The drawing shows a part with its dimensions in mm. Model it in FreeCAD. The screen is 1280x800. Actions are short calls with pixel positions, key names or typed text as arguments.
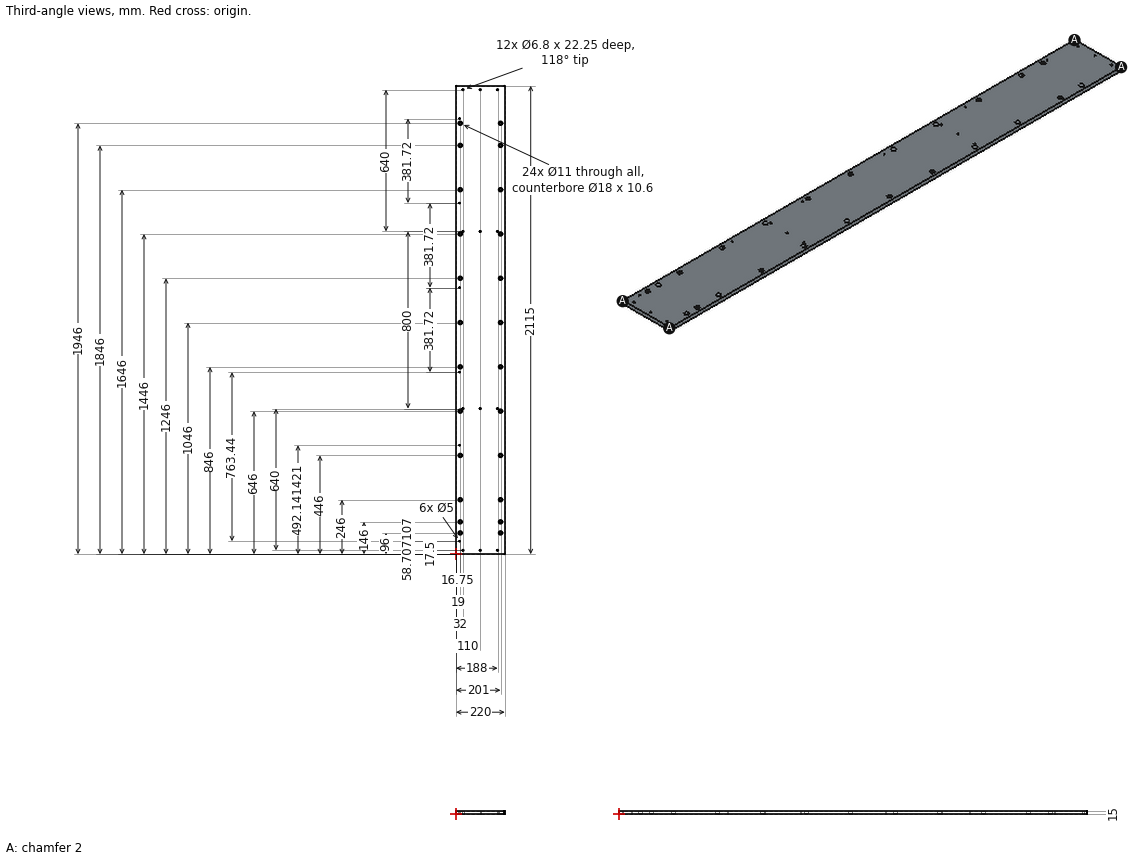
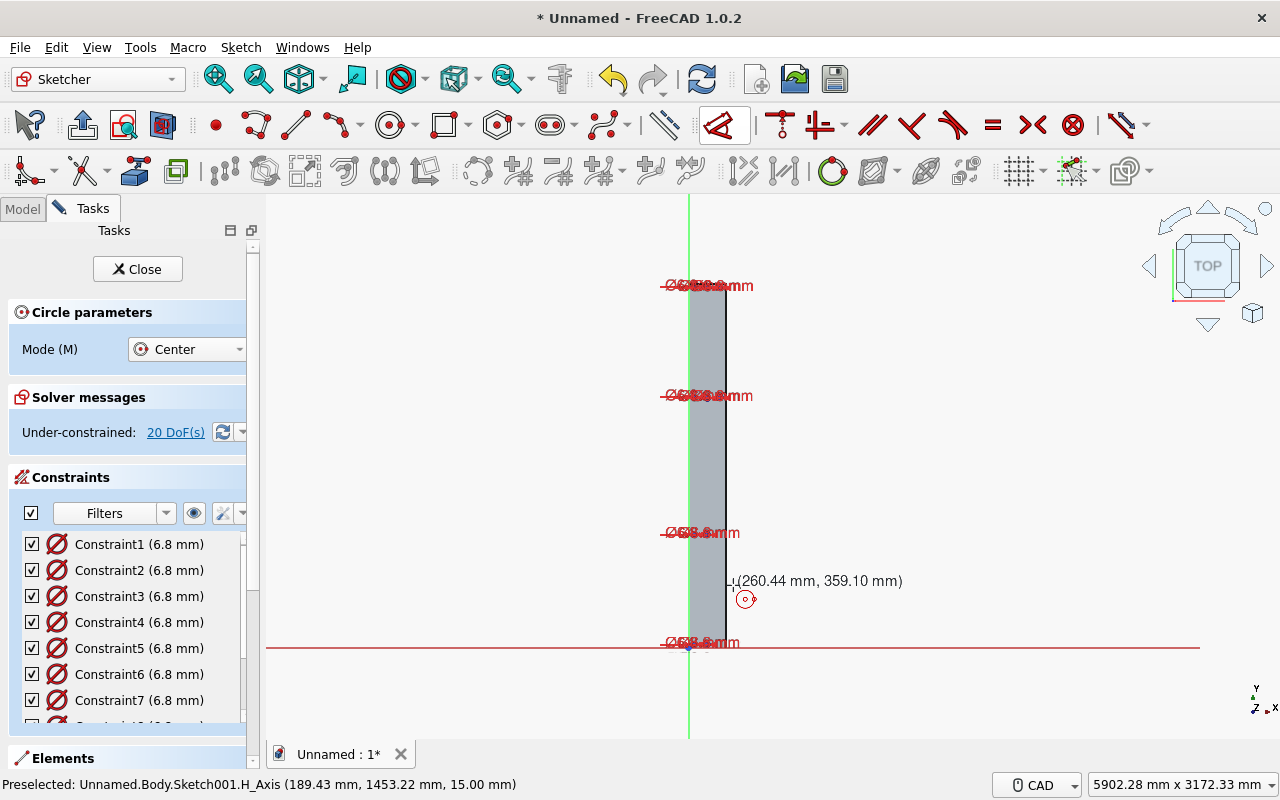
scroll(721, 535, up, 2)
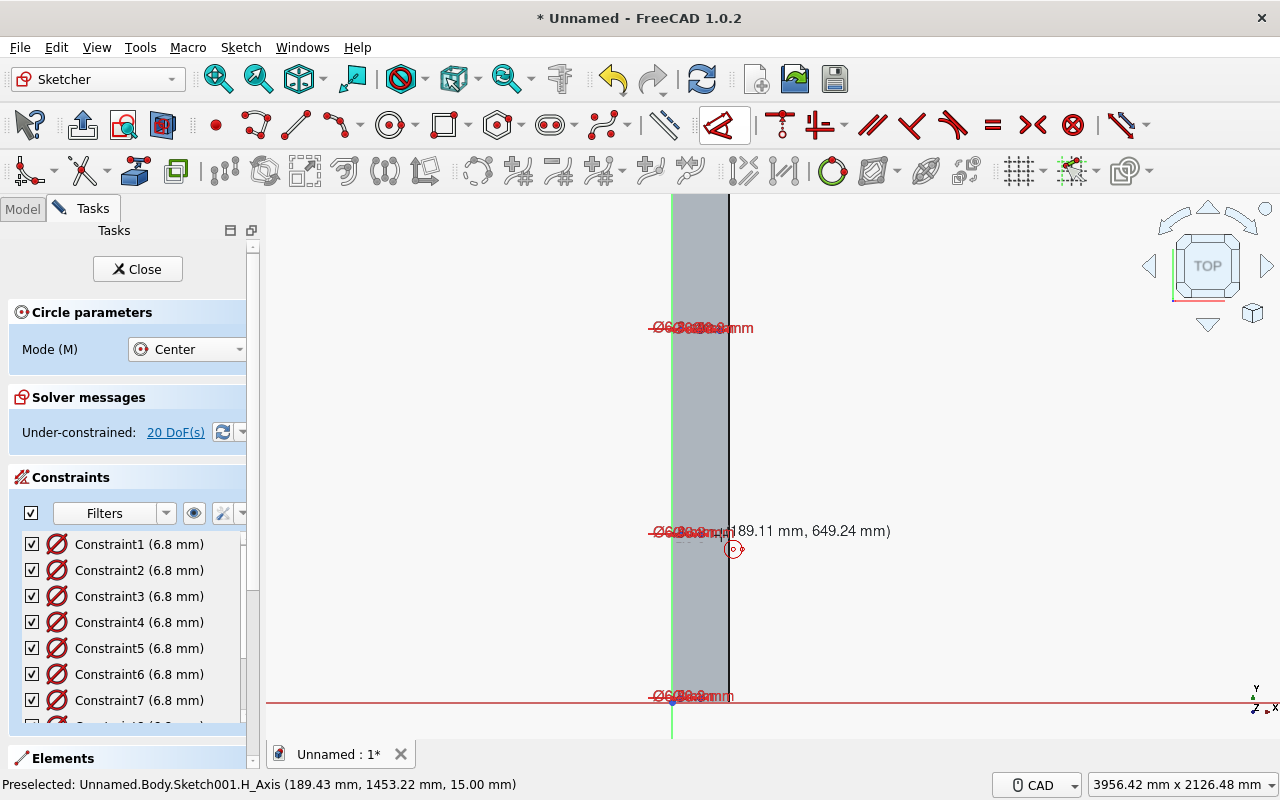
click(720, 534)
move(721, 533)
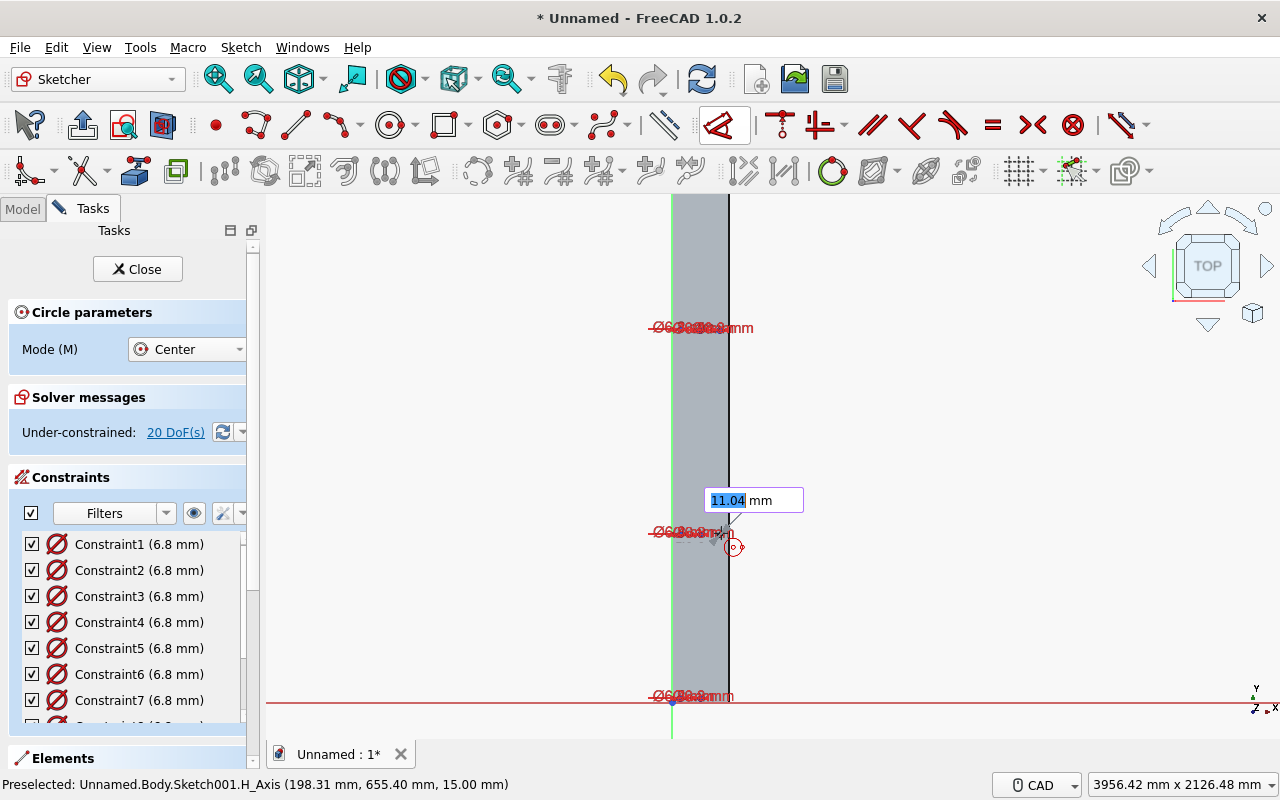
text(6.8)
key(Return)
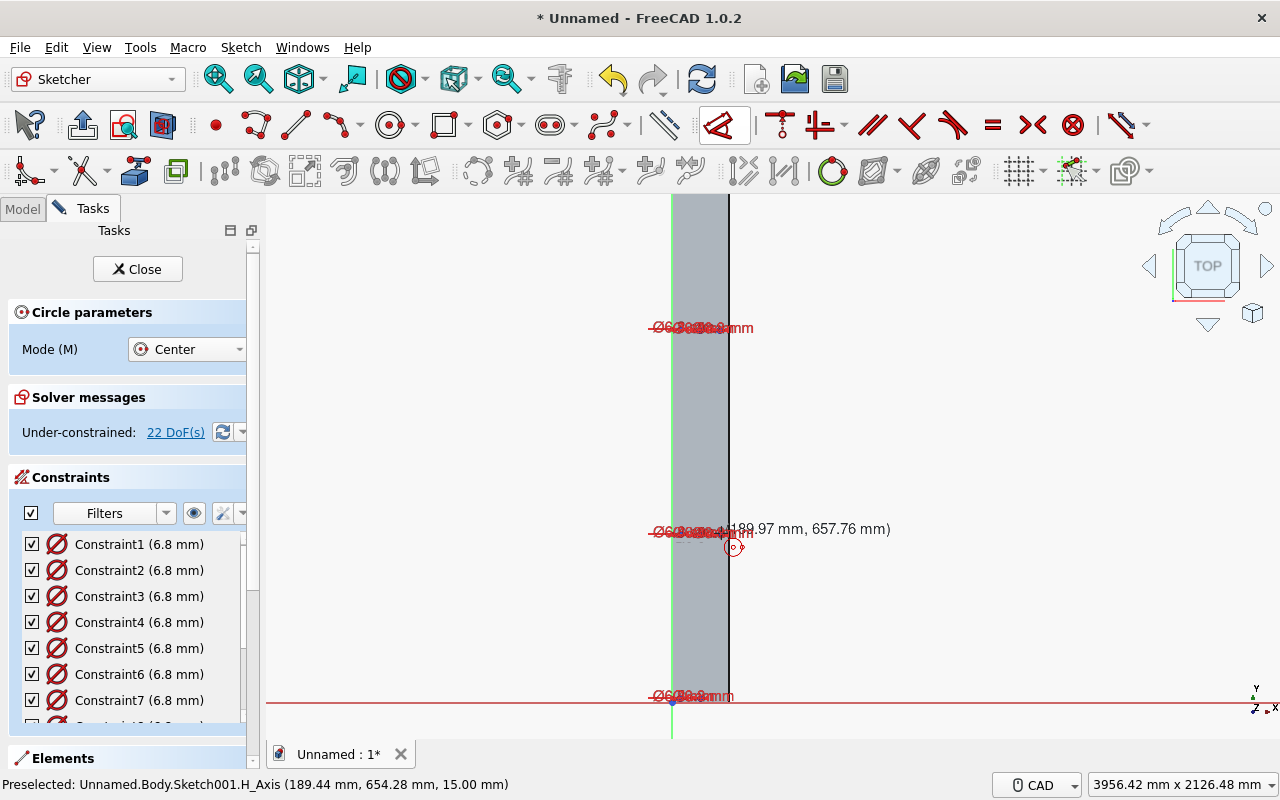
scroll(720, 698, up, 17)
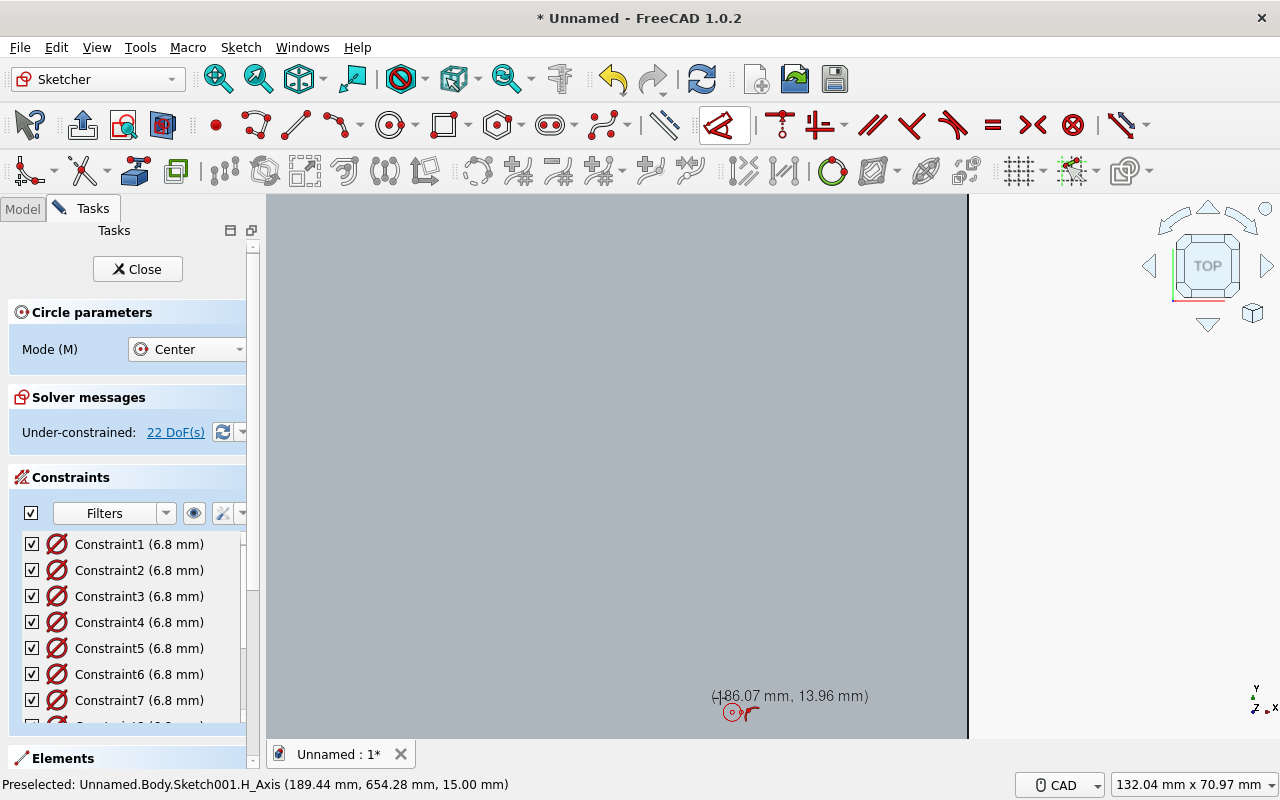
scroll(704, 466, down, 15)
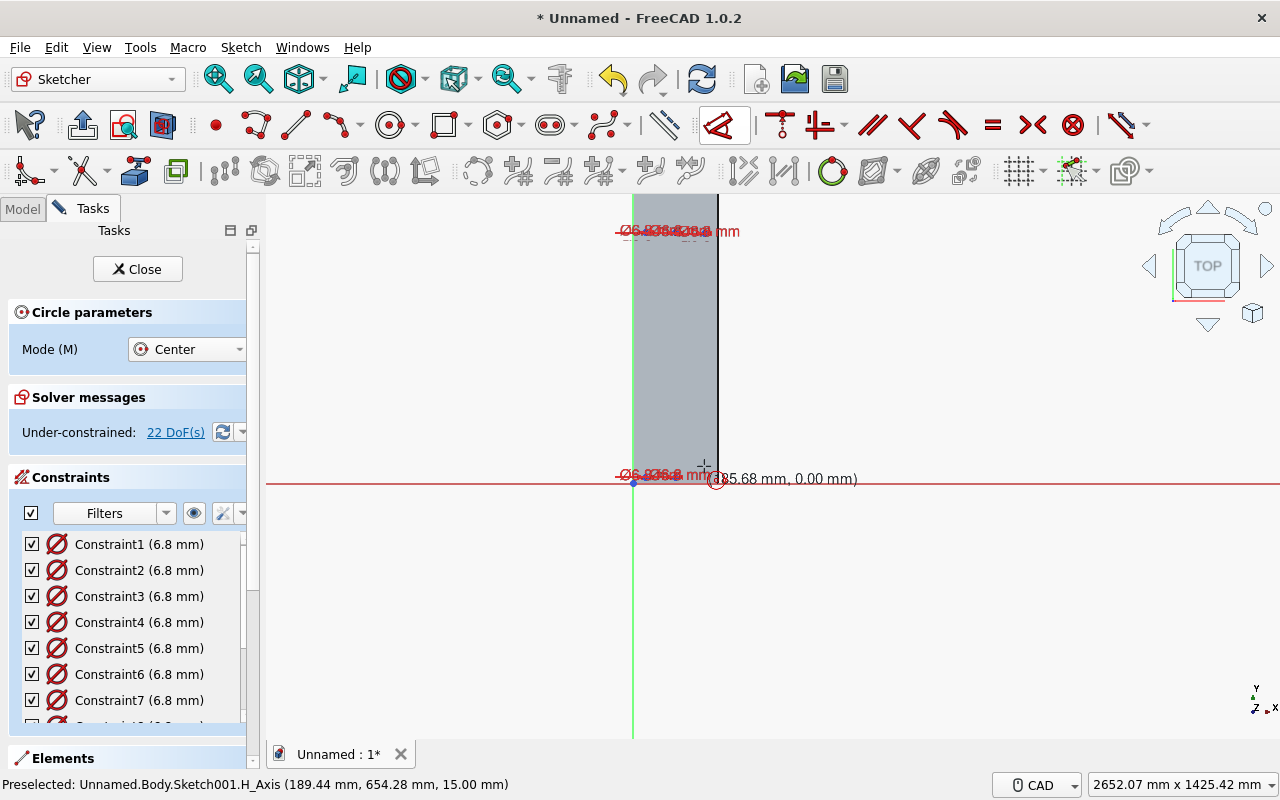
scroll(733, 711, down, 4)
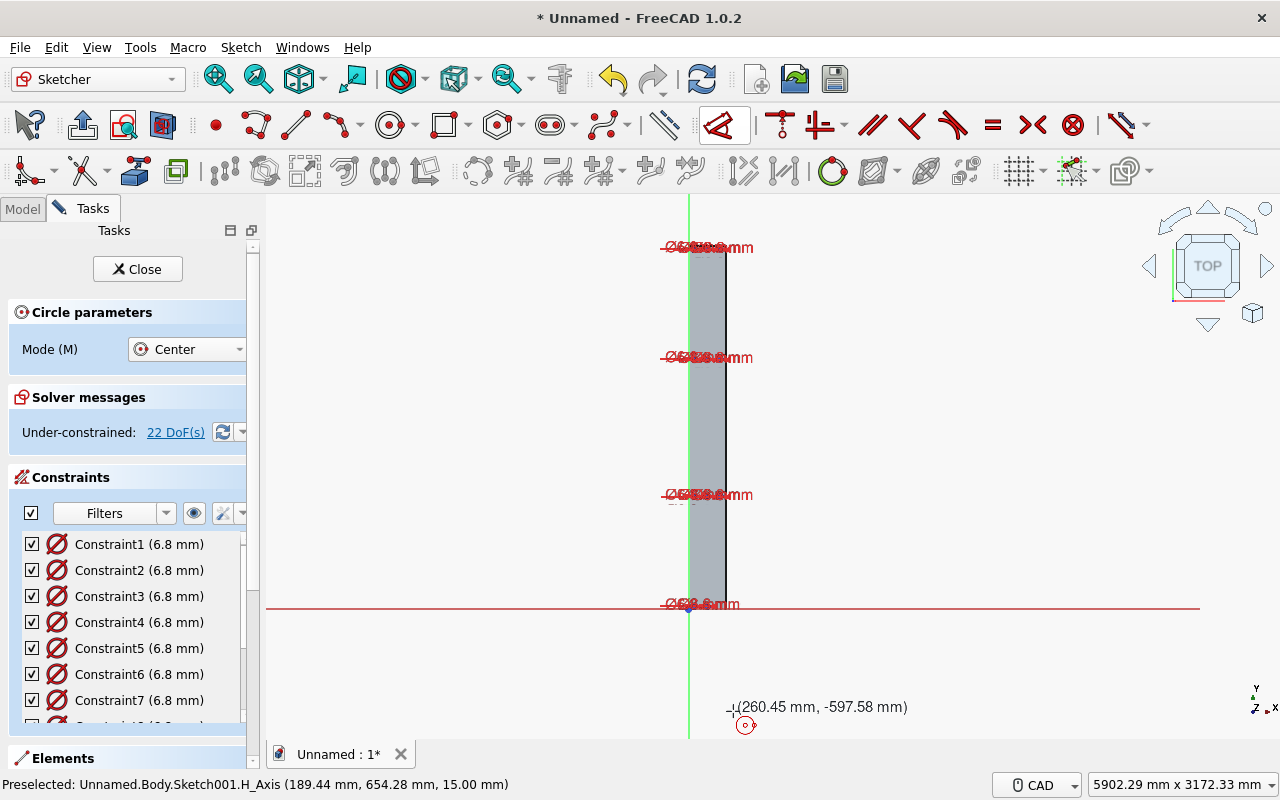
scroll(721, 606, up, 9)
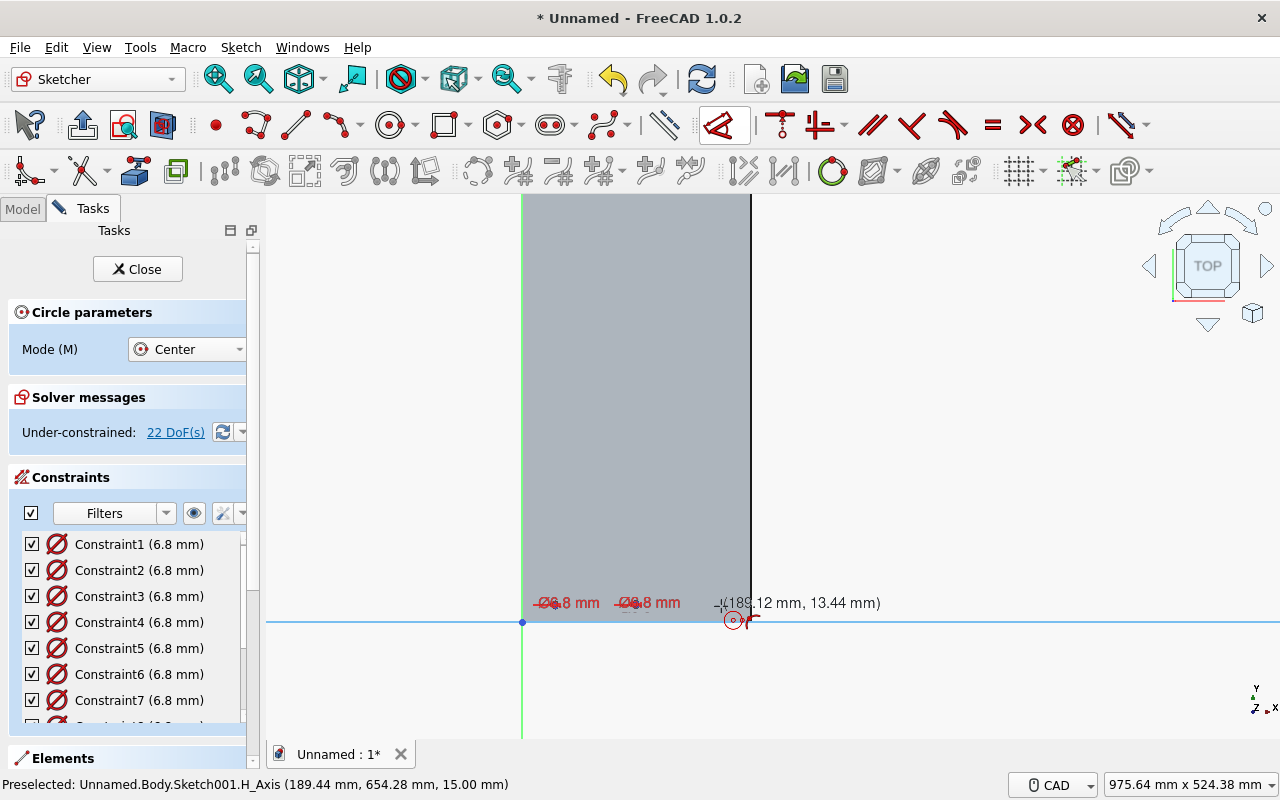
click(718, 604)
move(720, 602)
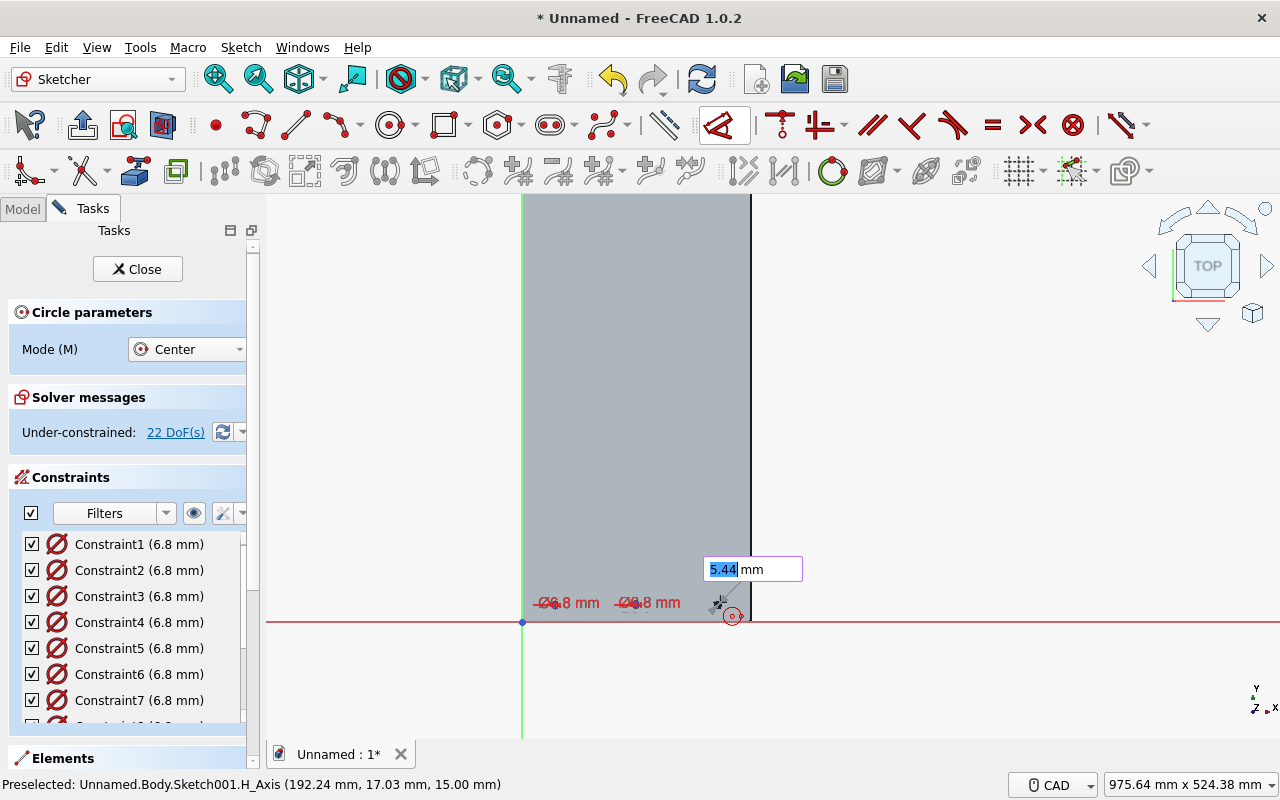
text(6.8)
key(Return)
key(Escape)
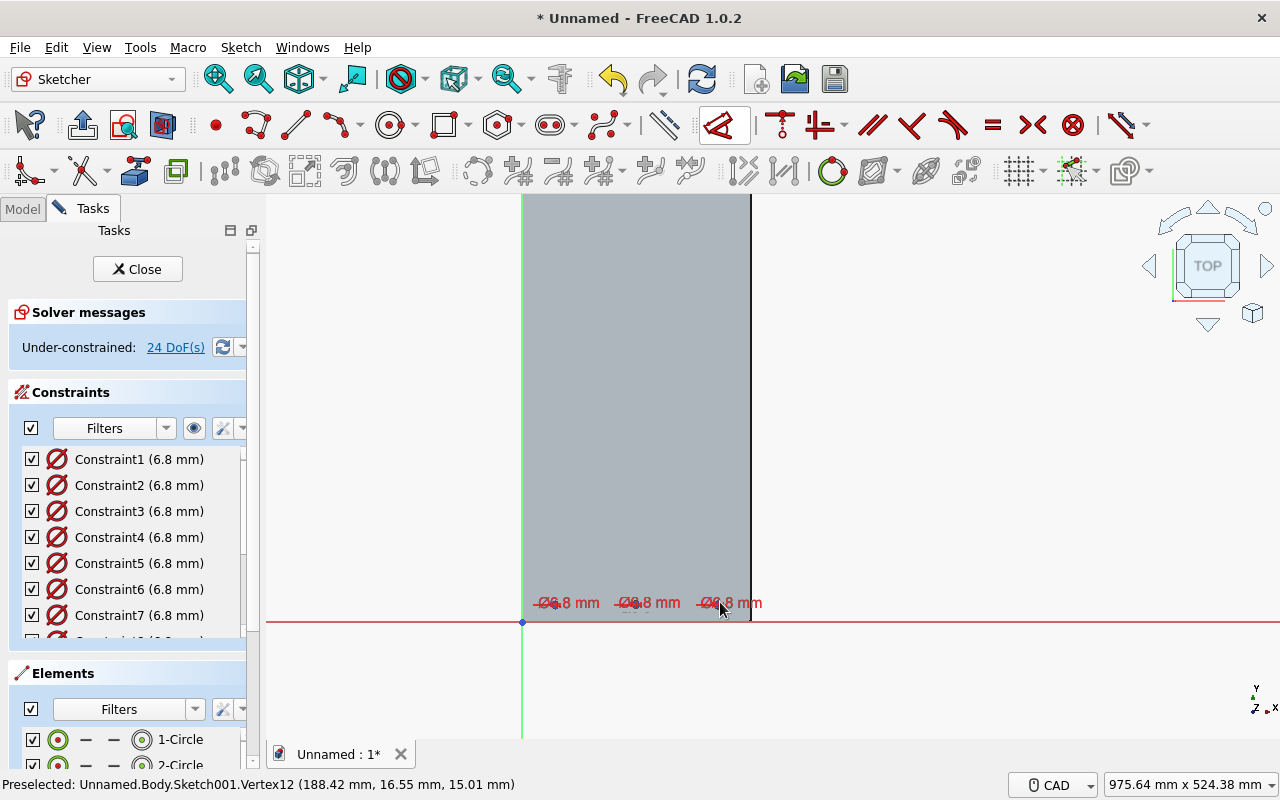
scroll(721, 652, down, 9)